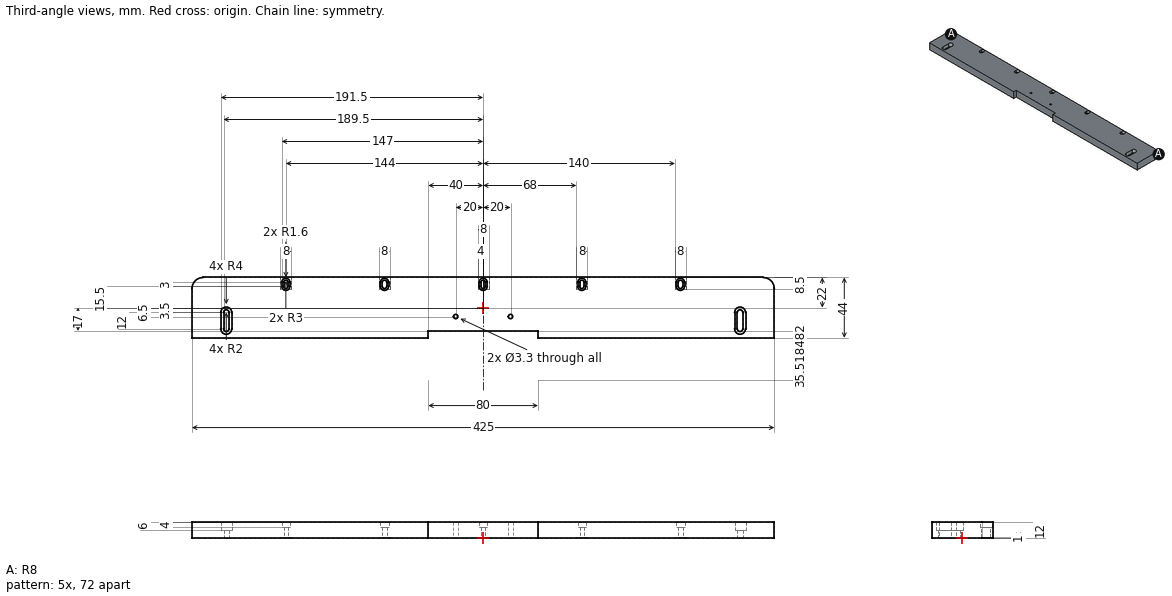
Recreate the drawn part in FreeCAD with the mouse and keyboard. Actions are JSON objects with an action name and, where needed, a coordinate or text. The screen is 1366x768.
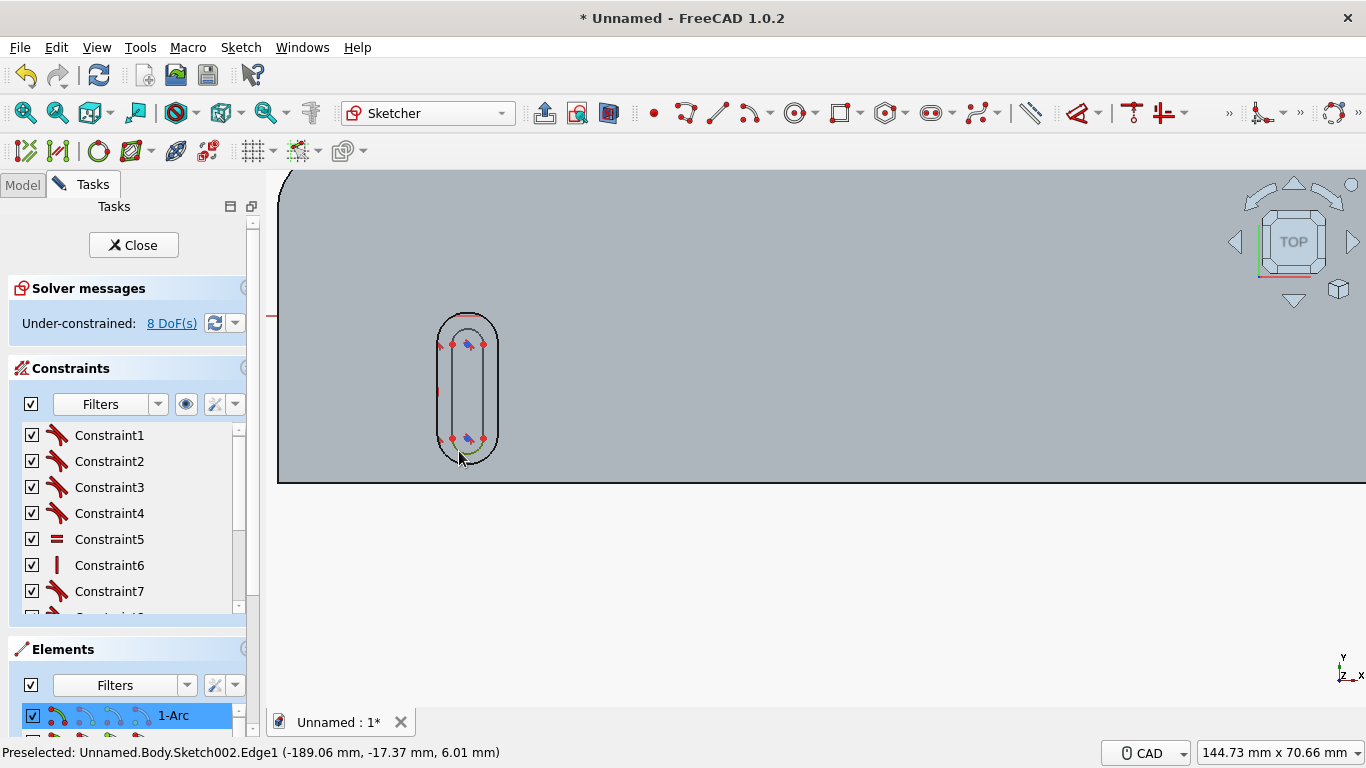
{"action": "scroll", "coordinate": [458, 453], "scroll_direction": "down", "scroll_amount": 8}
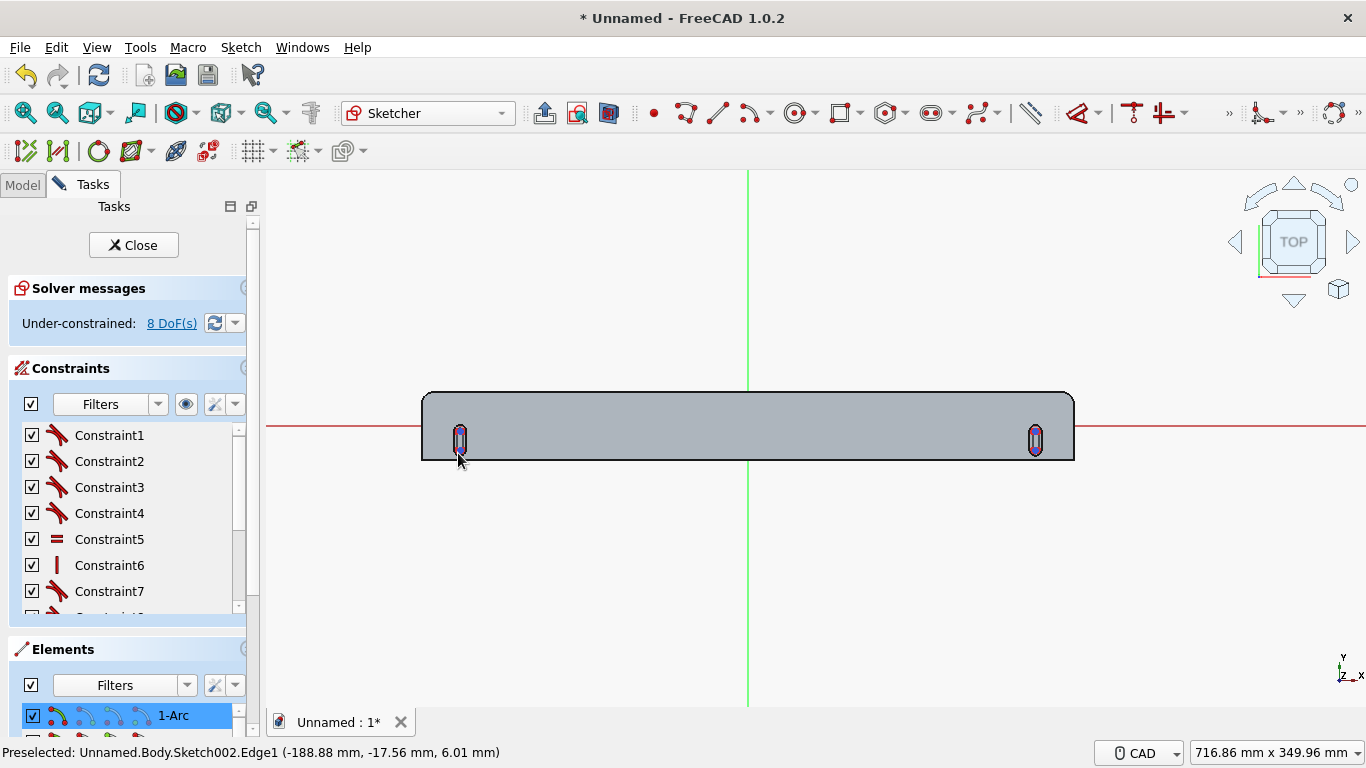
{"action": "scroll", "coordinate": [1034, 452], "scroll_direction": "up", "scroll_amount": 9}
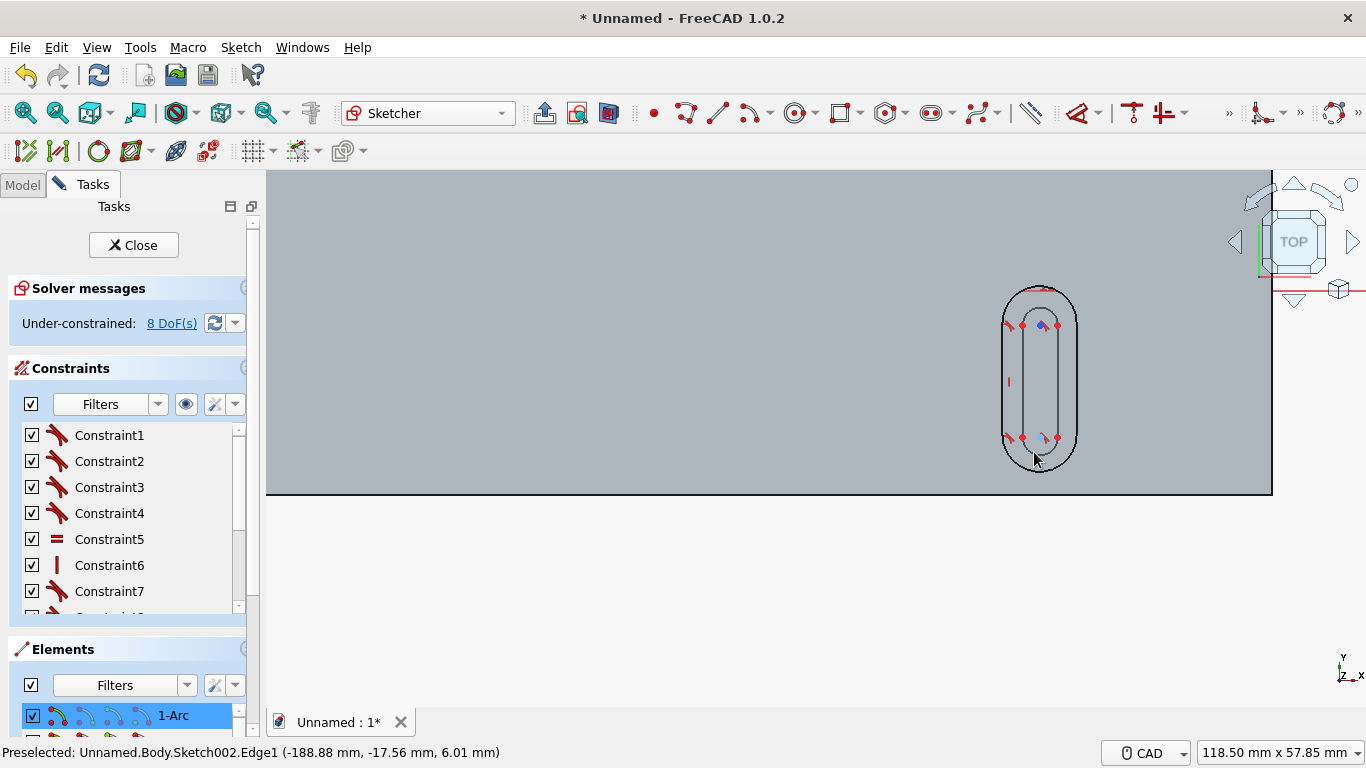
{"action": "left_click", "coordinate": [1030, 452]}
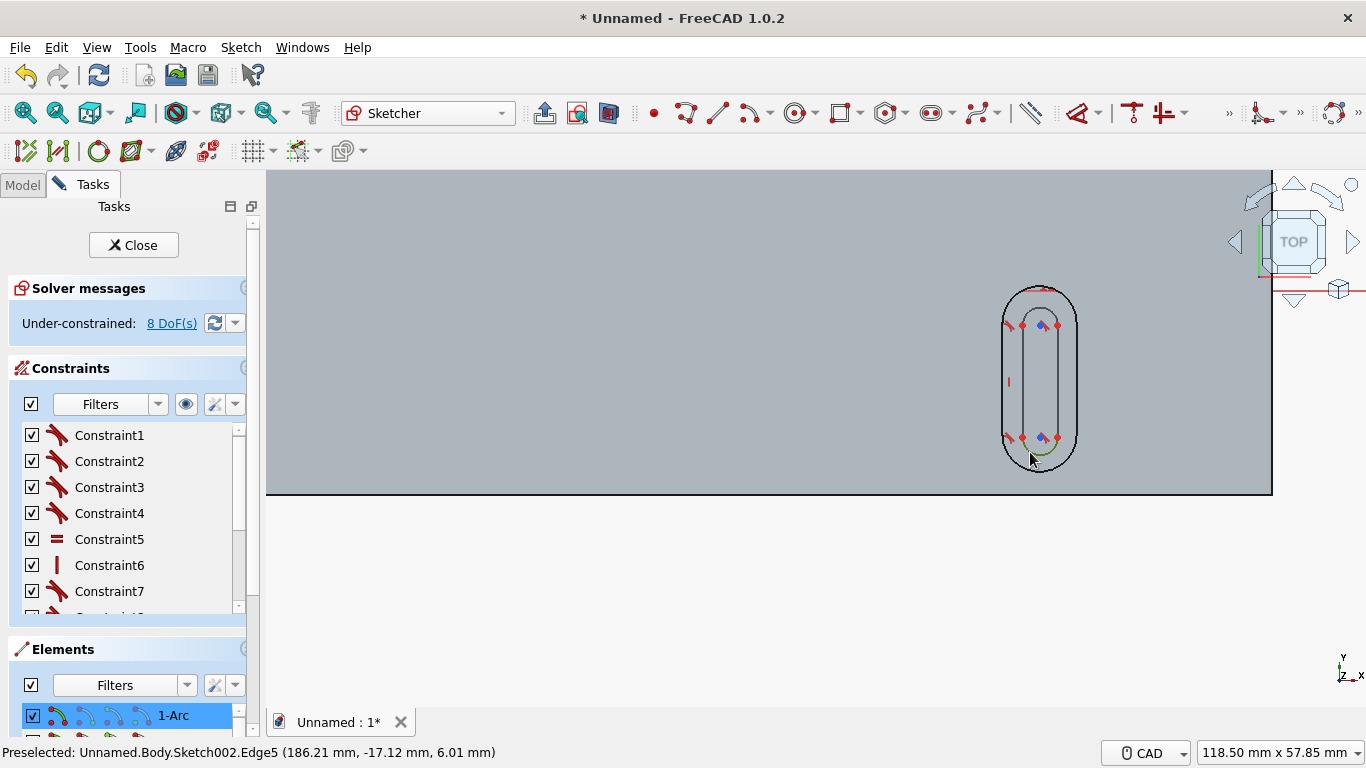
{"action": "key", "text": "e"}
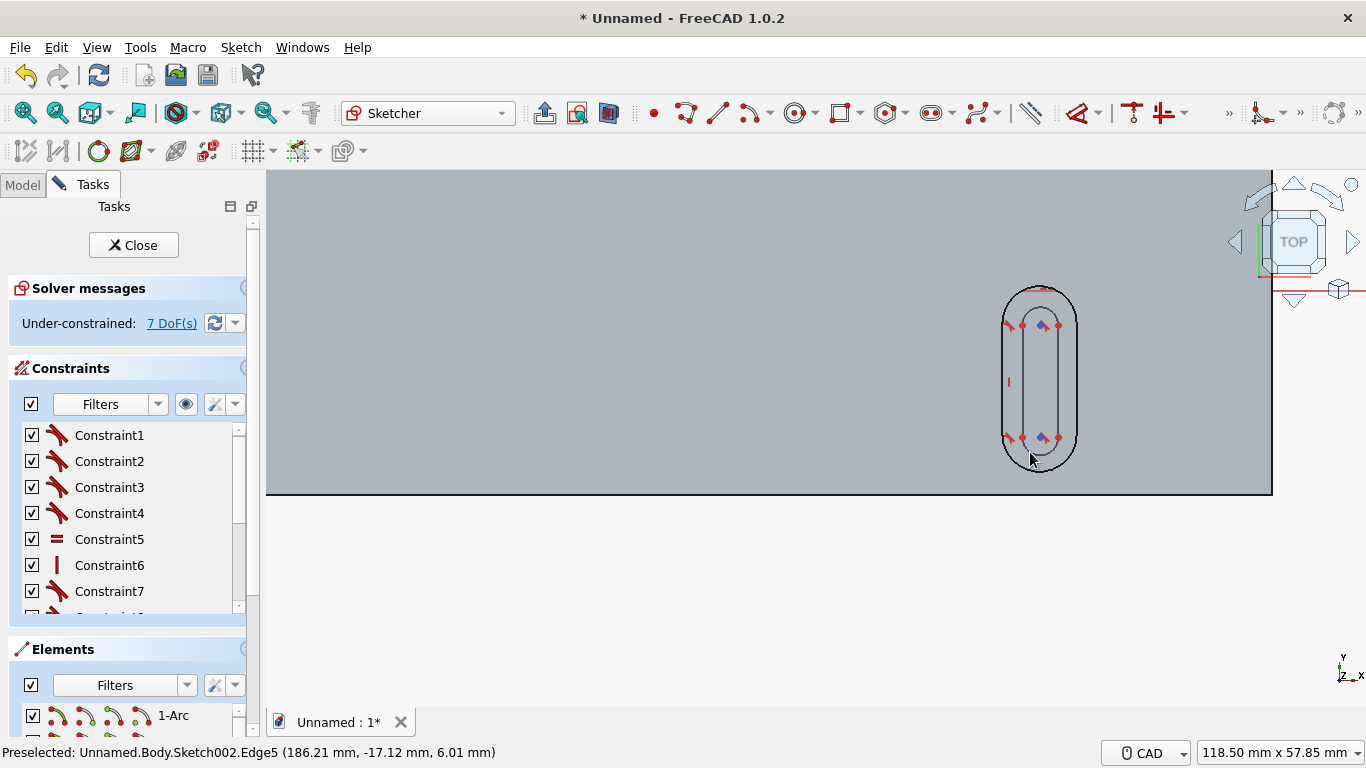
{"action": "scroll", "coordinate": [1034, 452], "scroll_direction": "down", "scroll_amount": 9}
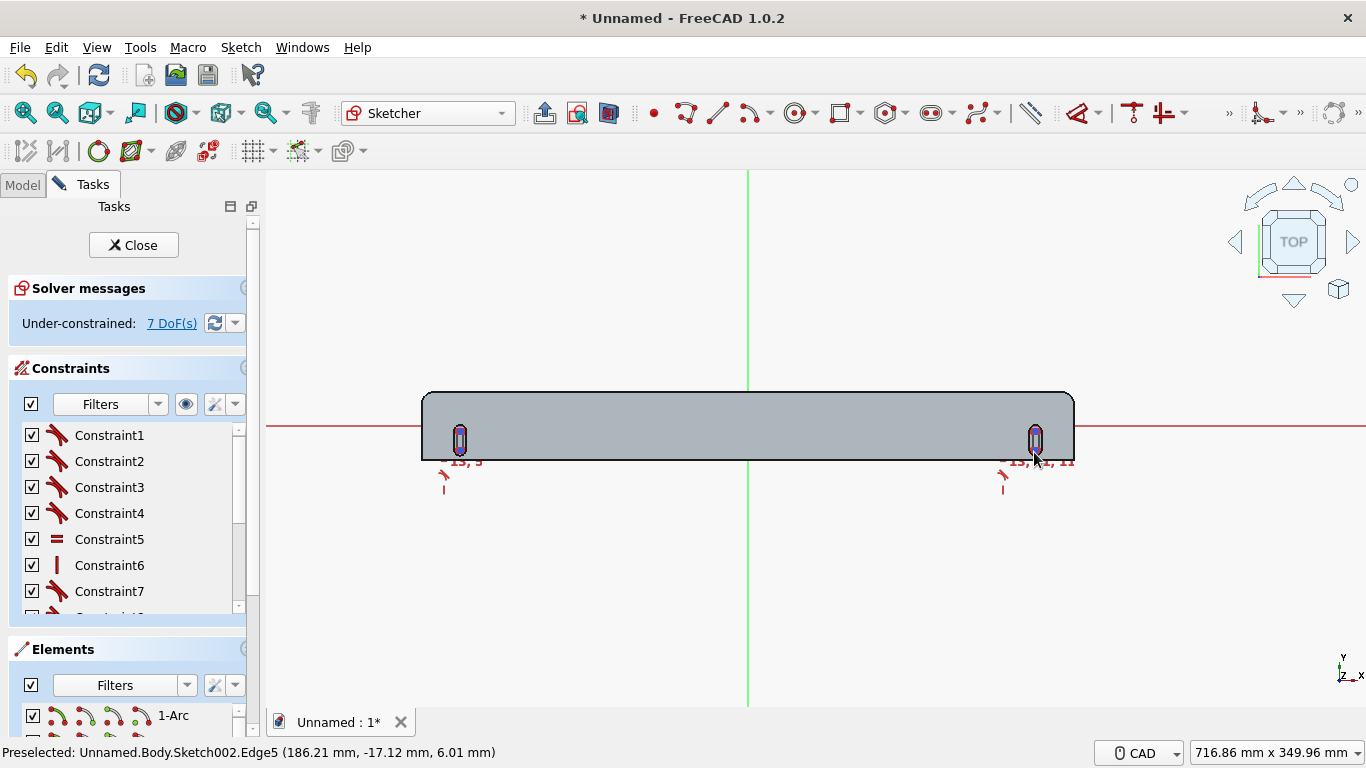
{"action": "scroll", "coordinate": [460, 450], "scroll_direction": "up", "scroll_amount": 8}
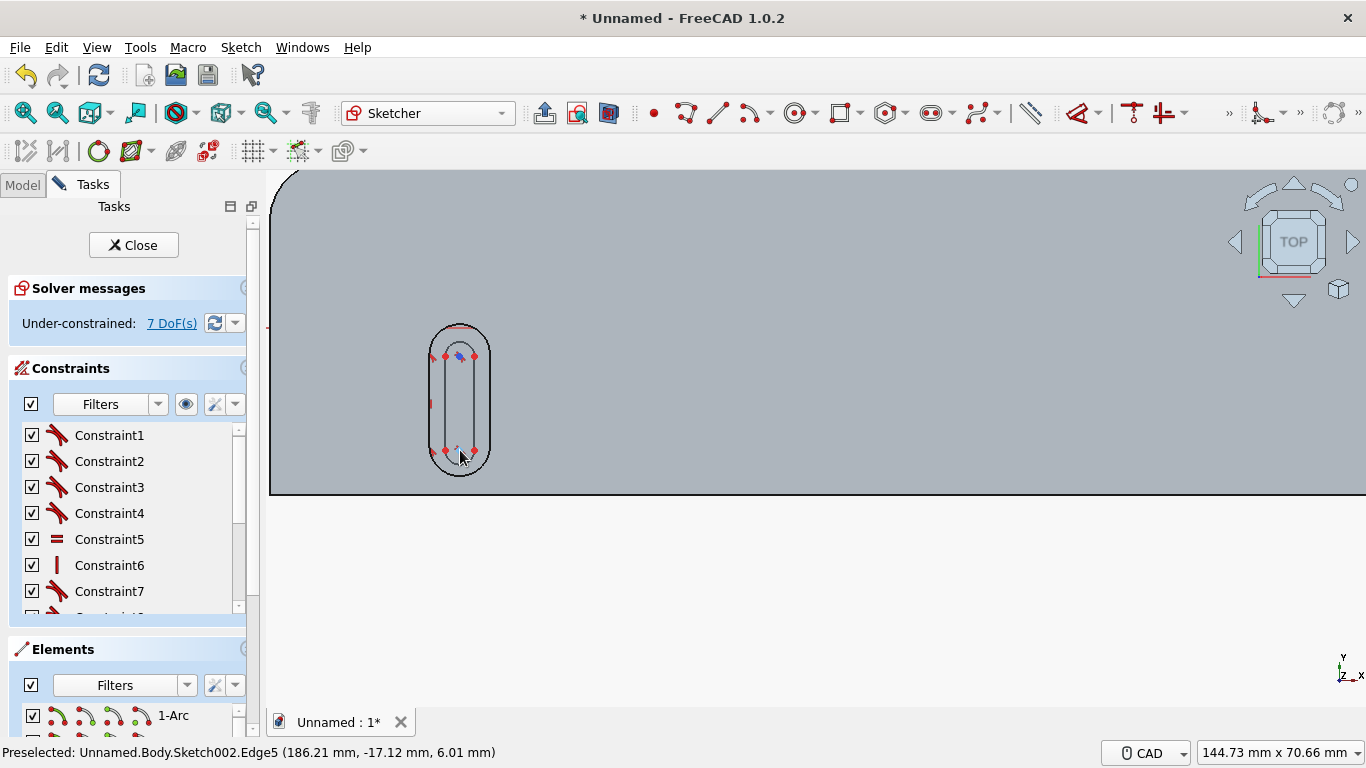
{"action": "left_click", "coordinate": [460, 450]}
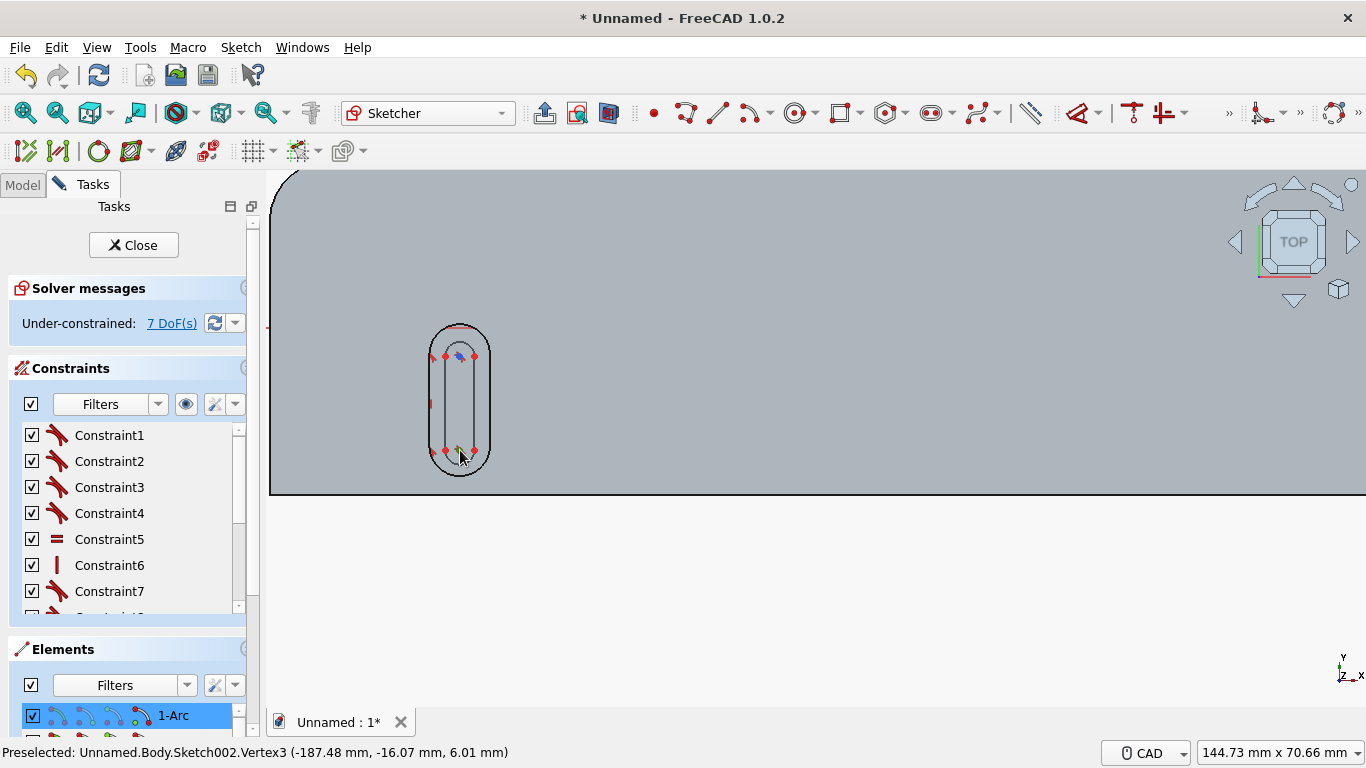
{"action": "scroll", "coordinate": [460, 450], "scroll_direction": "down", "scroll_amount": 8}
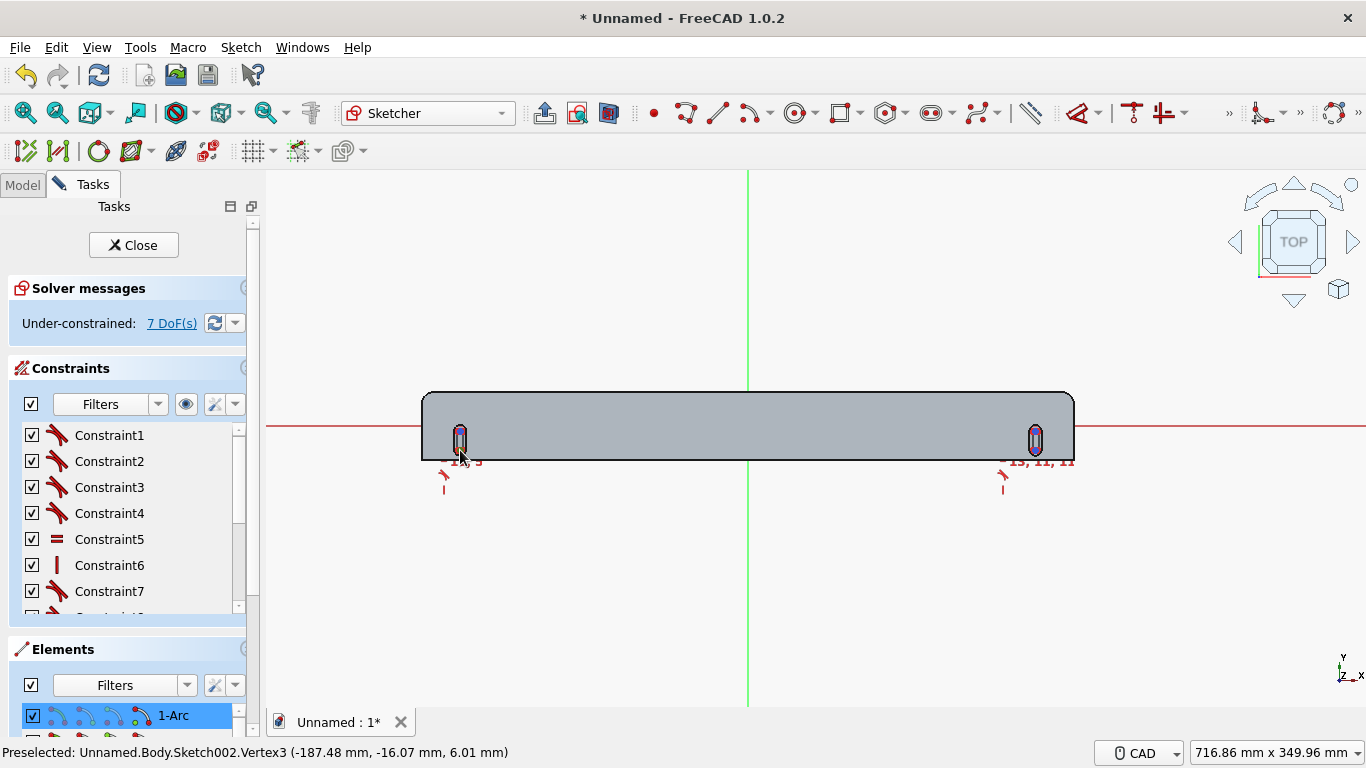
{"action": "scroll", "coordinate": [1036, 450], "scroll_direction": "up", "scroll_amount": 8}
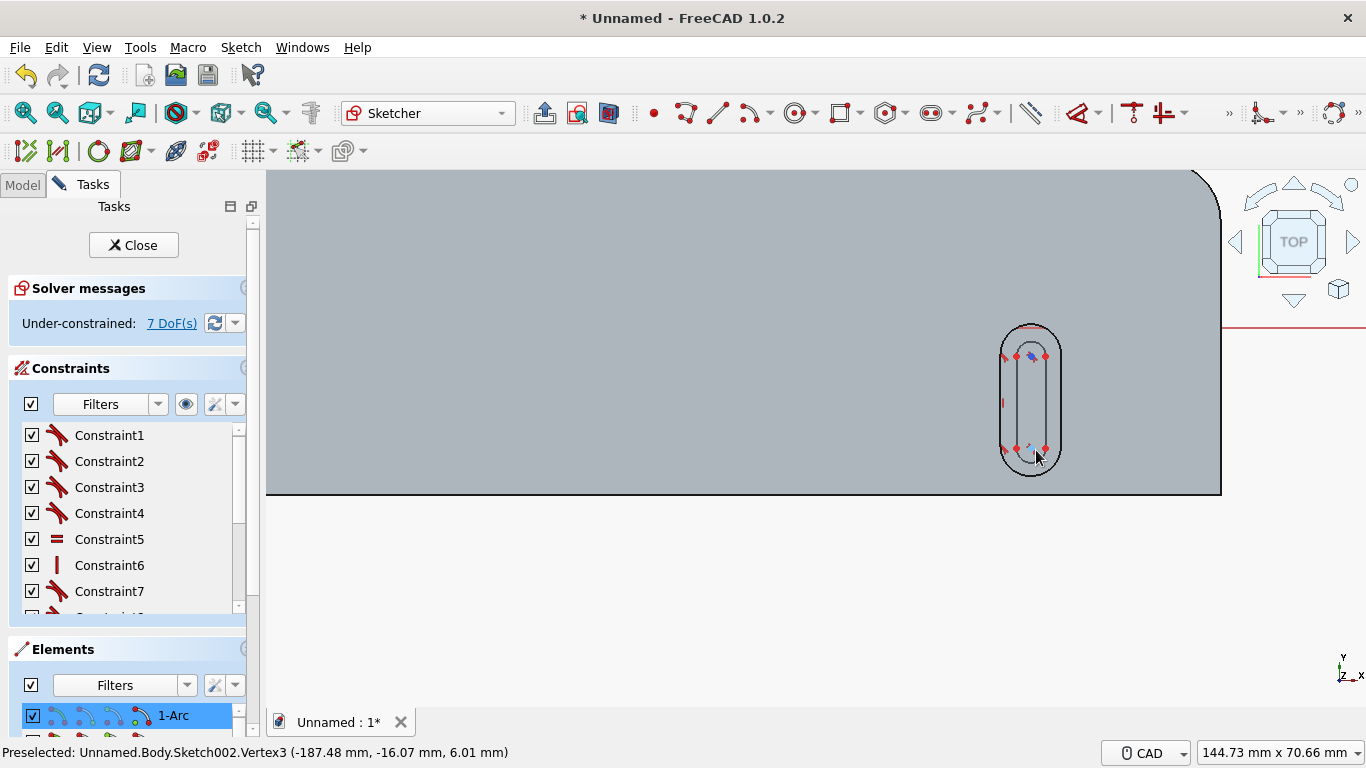
{"action": "left_click", "coordinate": [1031, 448]}